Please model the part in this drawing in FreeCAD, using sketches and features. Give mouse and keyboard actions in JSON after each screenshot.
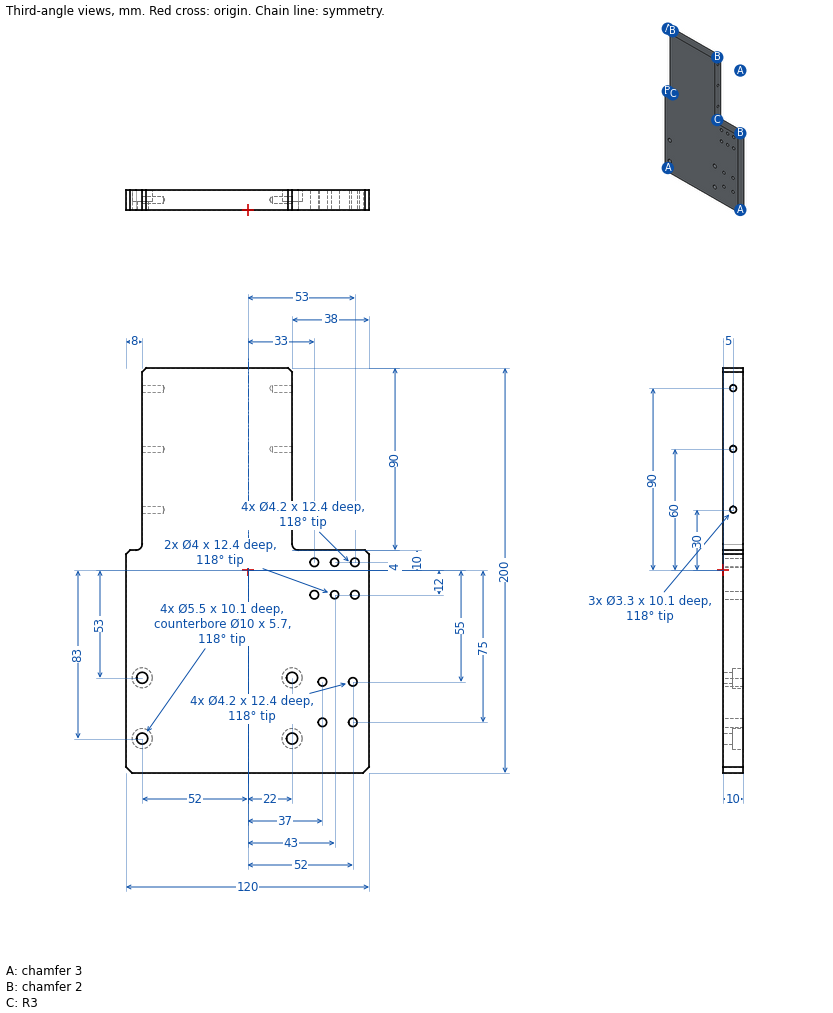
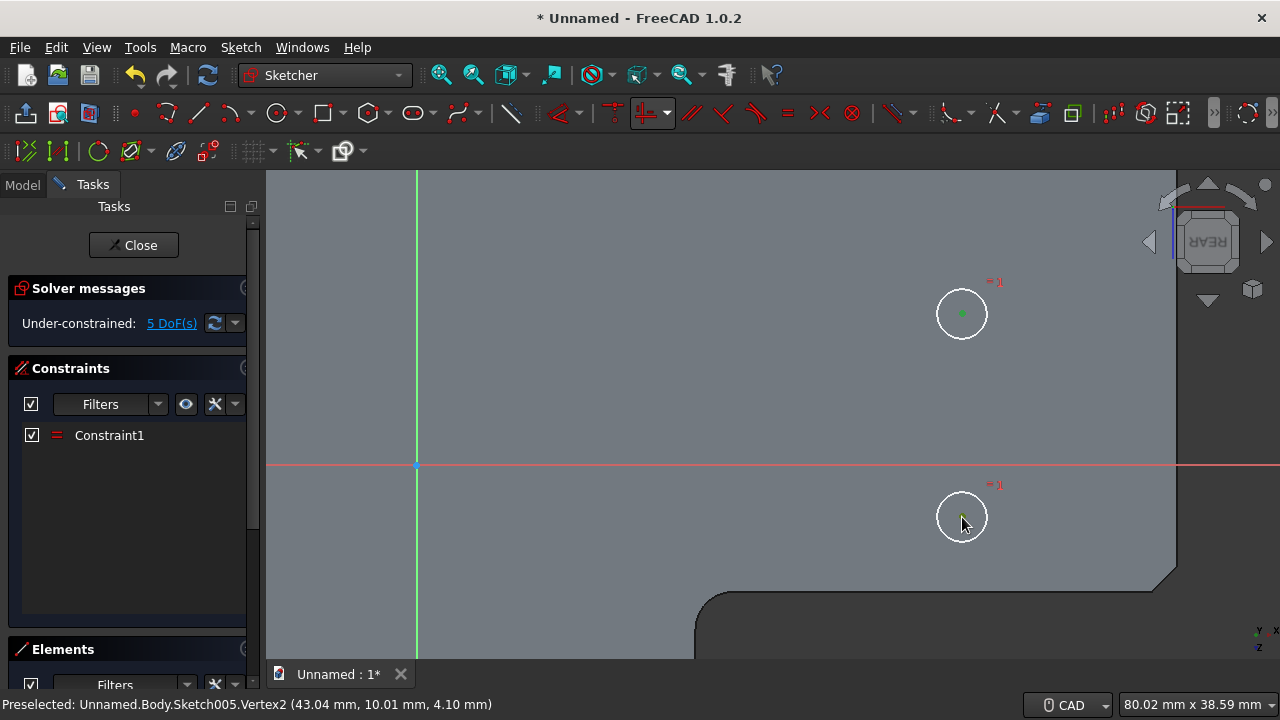
{"action": "left_click", "coordinate": [670, 114]}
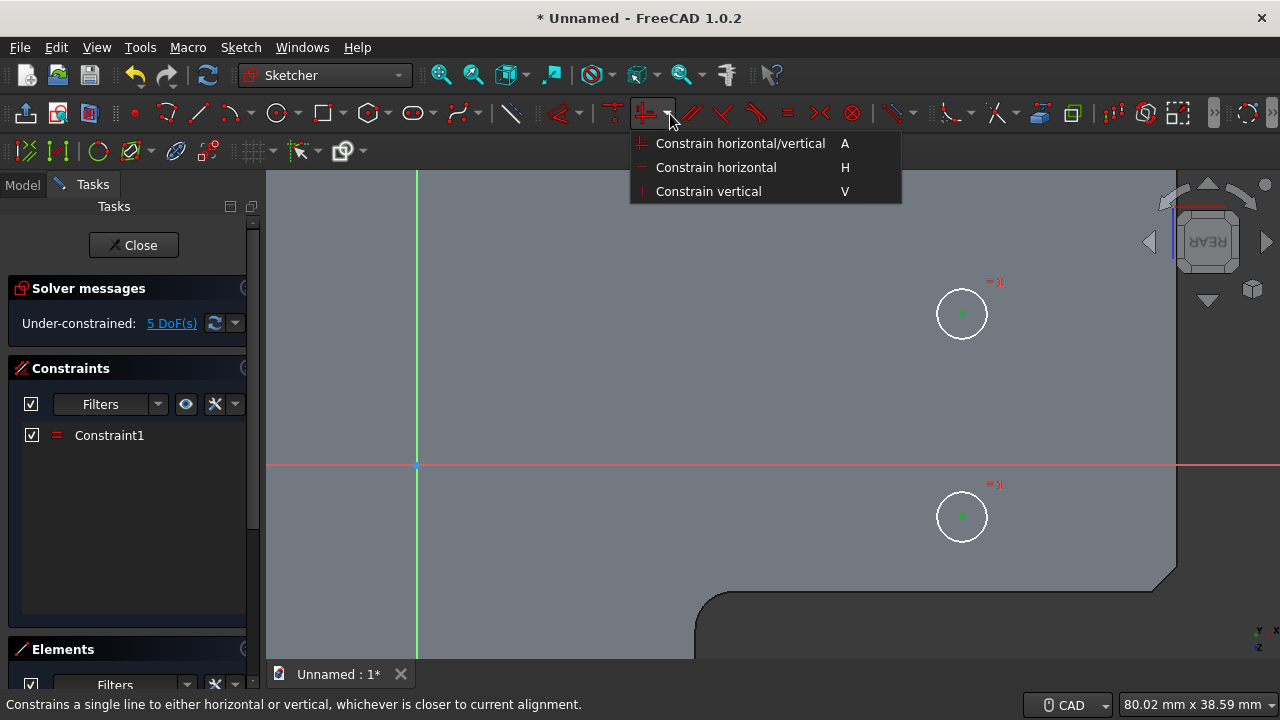
{"action": "left_click", "coordinate": [766, 191]}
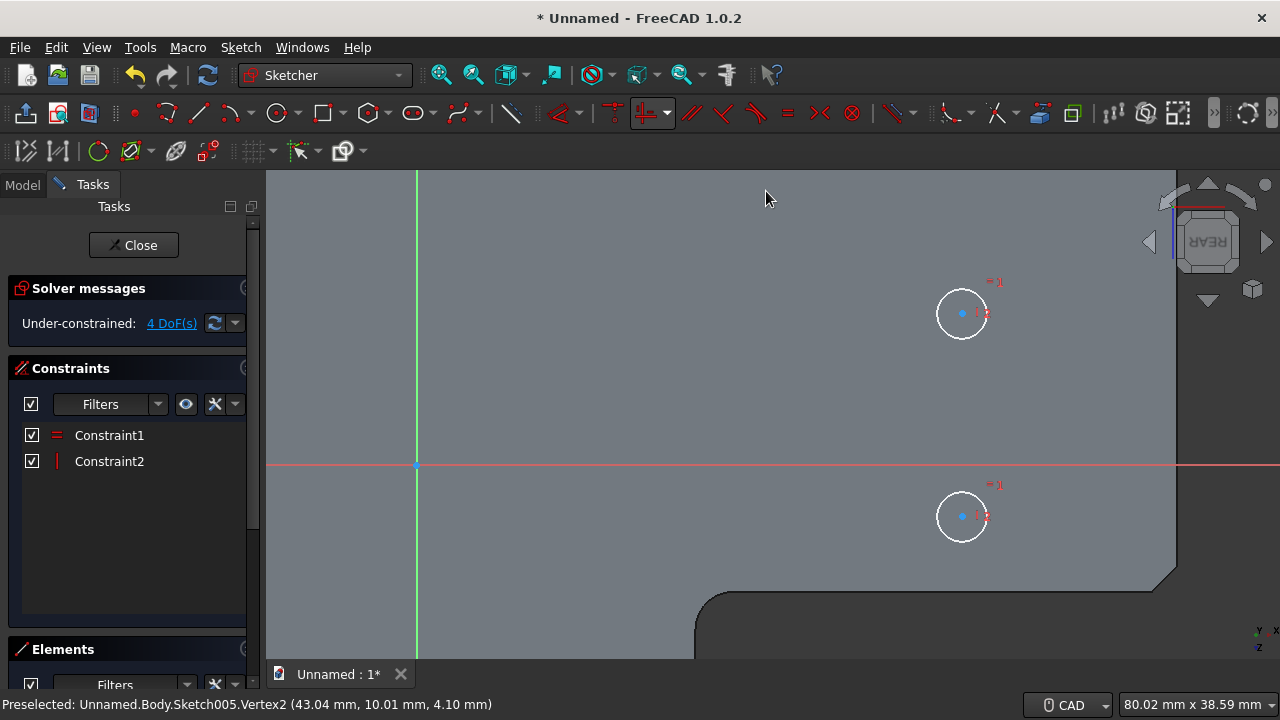
{"action": "left_click", "coordinate": [558, 114]}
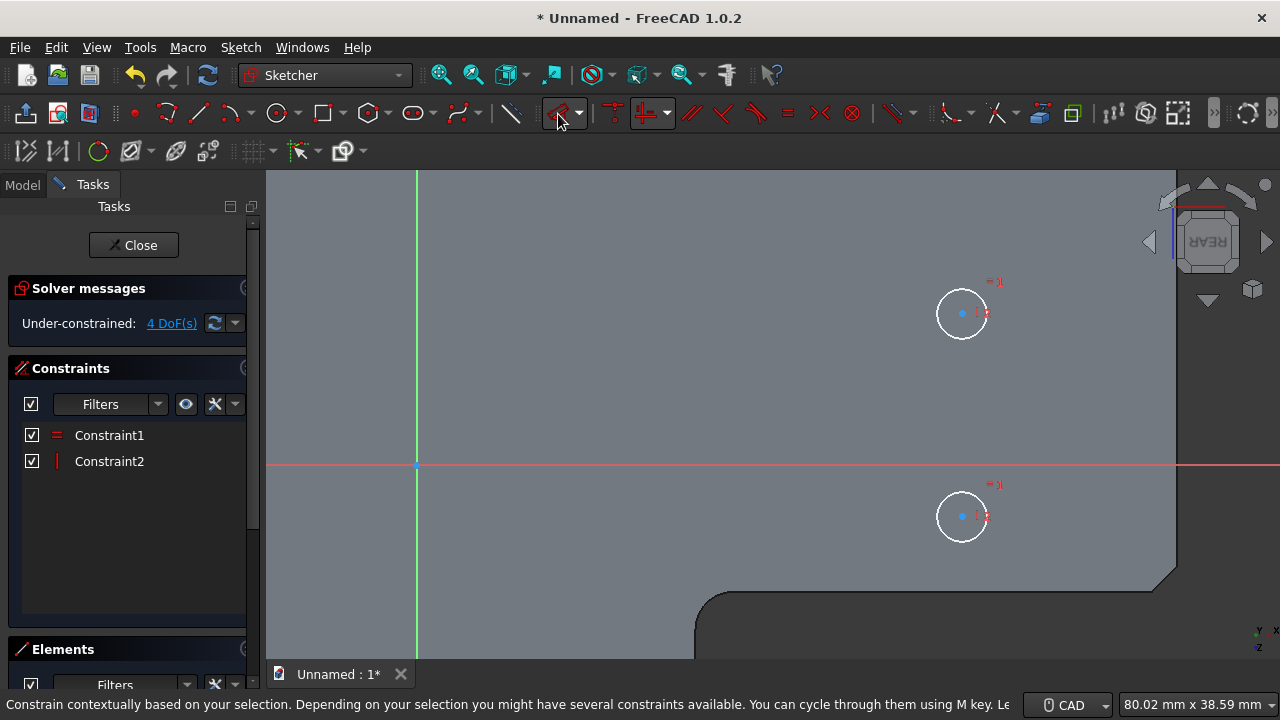
{"action": "left_click", "coordinate": [979, 296]}
{"action": "left_click", "coordinate": [1001, 273]}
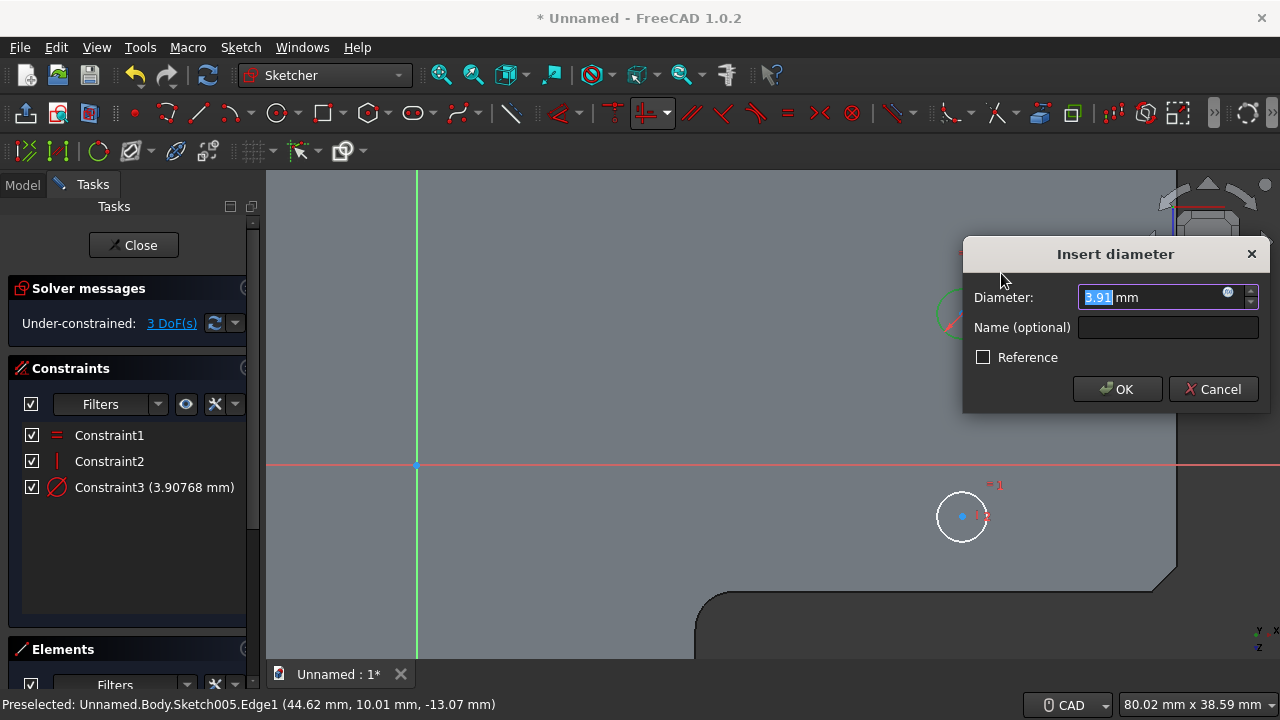
{"action": "type", "text": "4"}
{"action": "key", "text": "Return"}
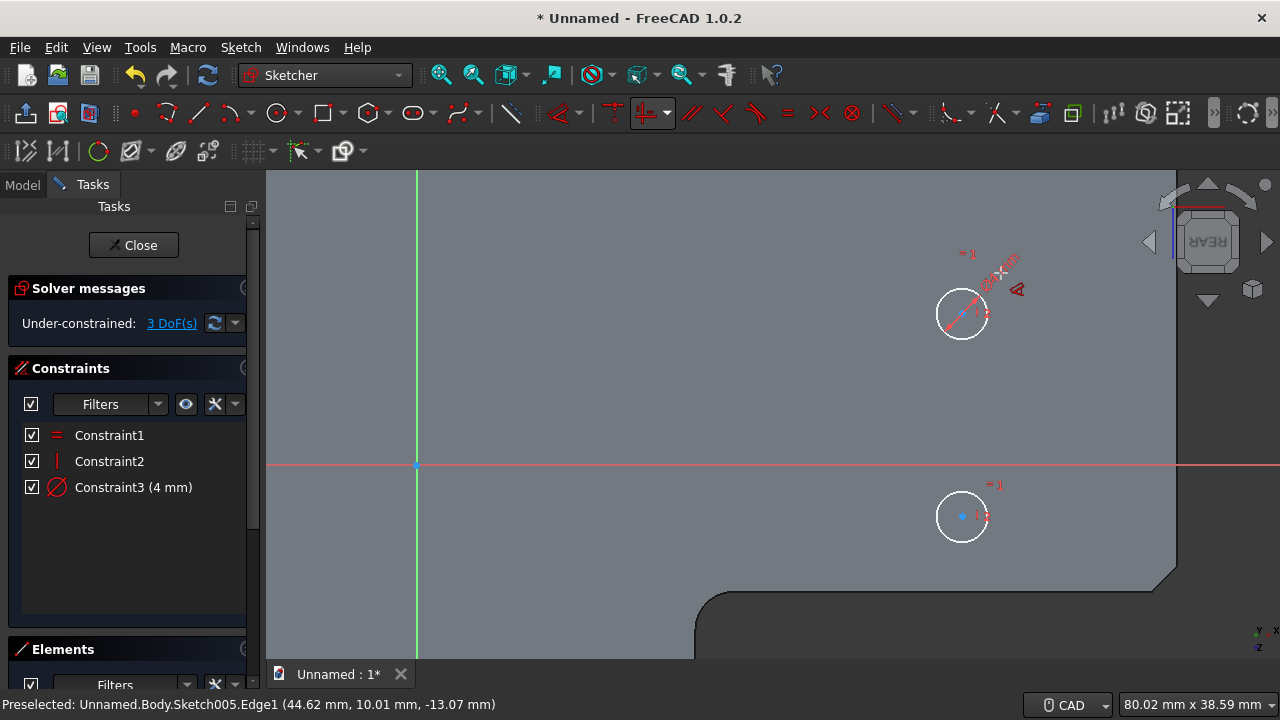
{"action": "left_click", "coordinate": [962, 517]}
{"action": "left_click", "coordinate": [383, 491]}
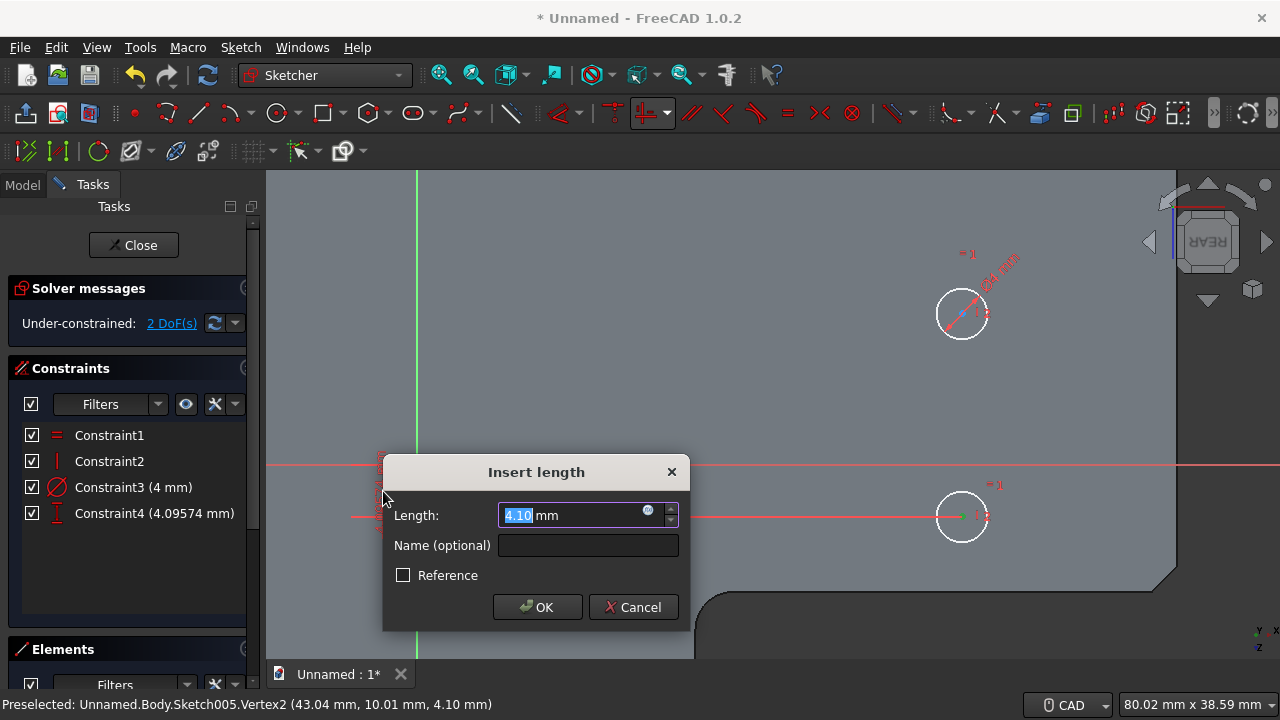
{"action": "type", "text": "4"}
{"action": "key", "text": "Return"}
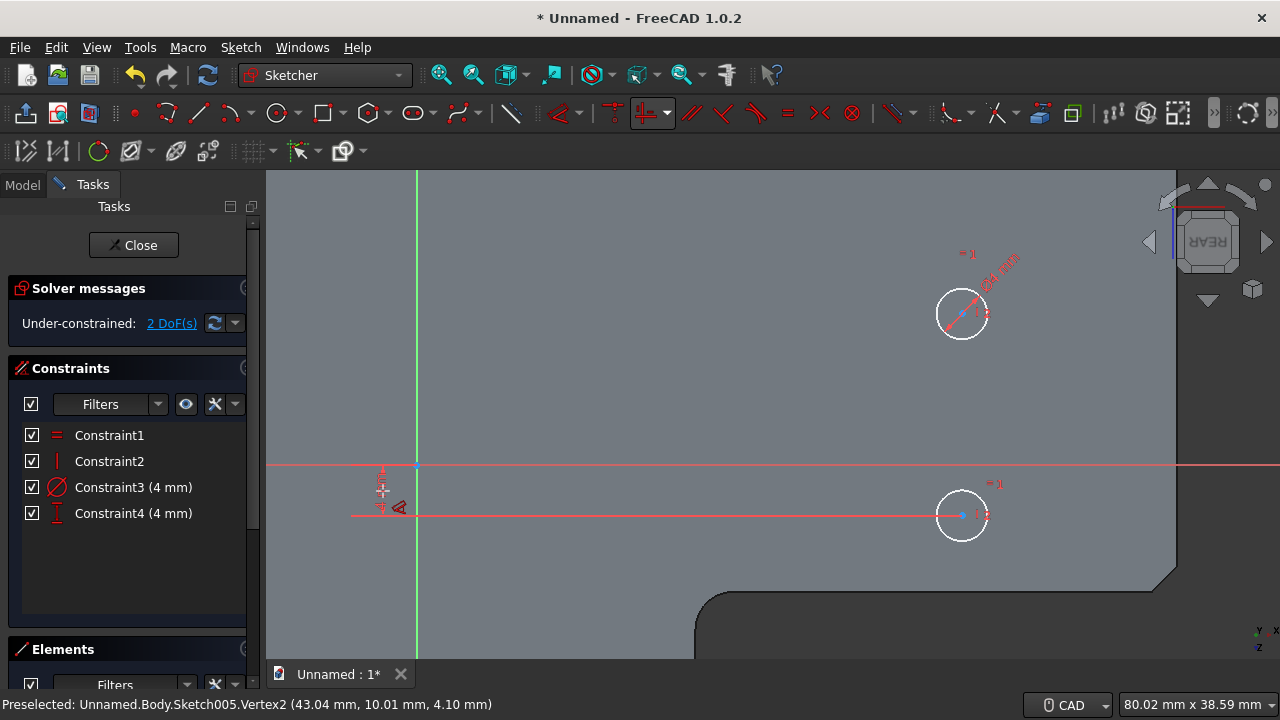
{"action": "left_click", "coordinate": [962, 314]}
{"action": "left_click", "coordinate": [689, 280]}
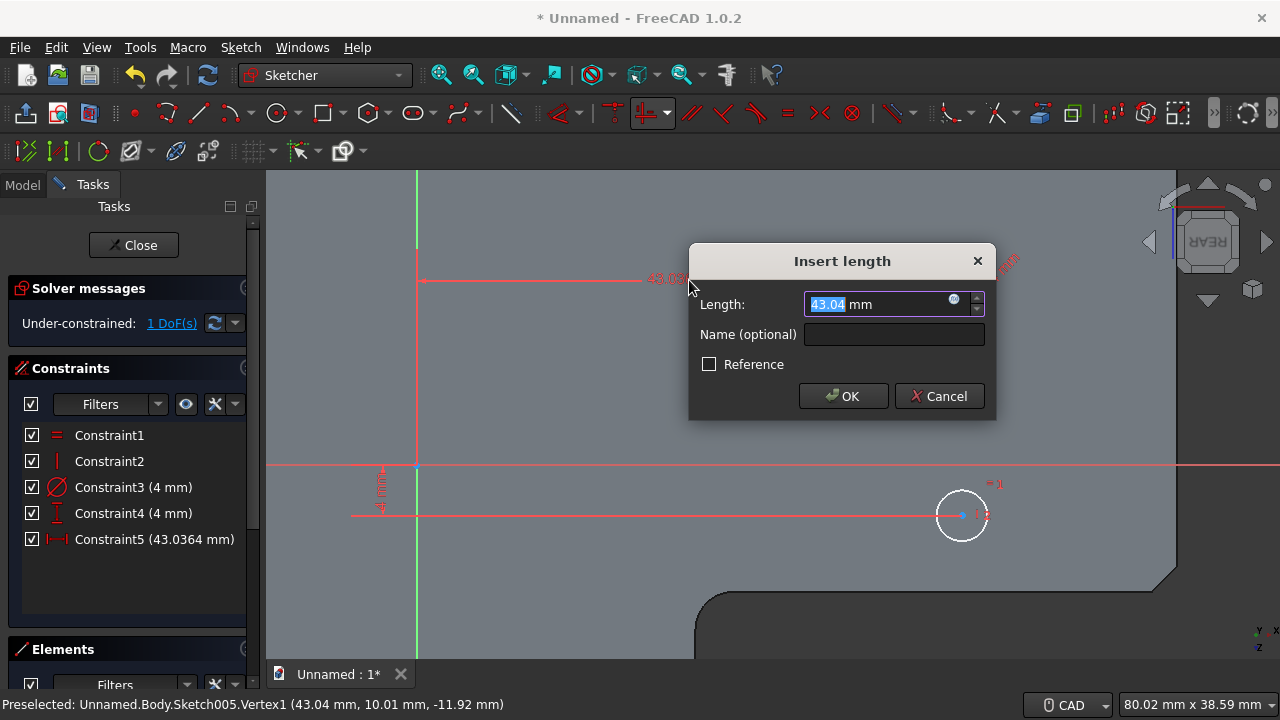
{"action": "type", "text": "43"}
{"action": "key", "text": "Return"}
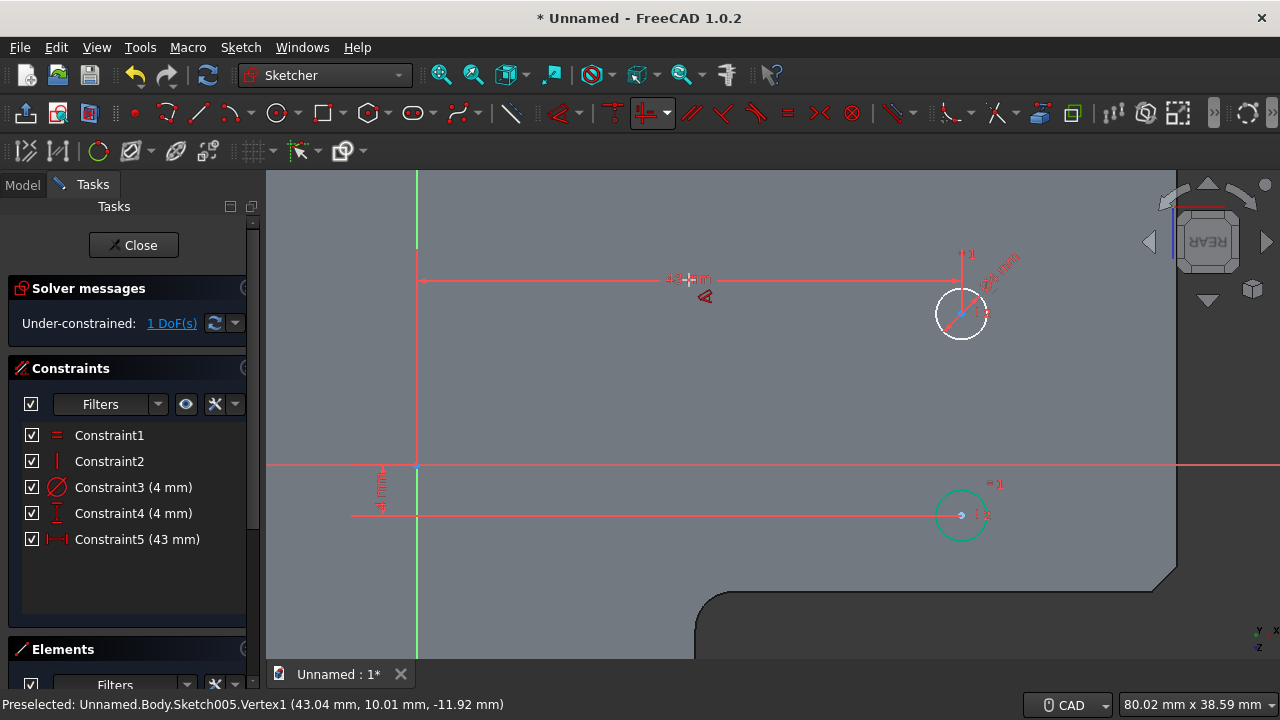
{"action": "left_click", "coordinate": [962, 314]}
{"action": "left_click", "coordinate": [383, 390]}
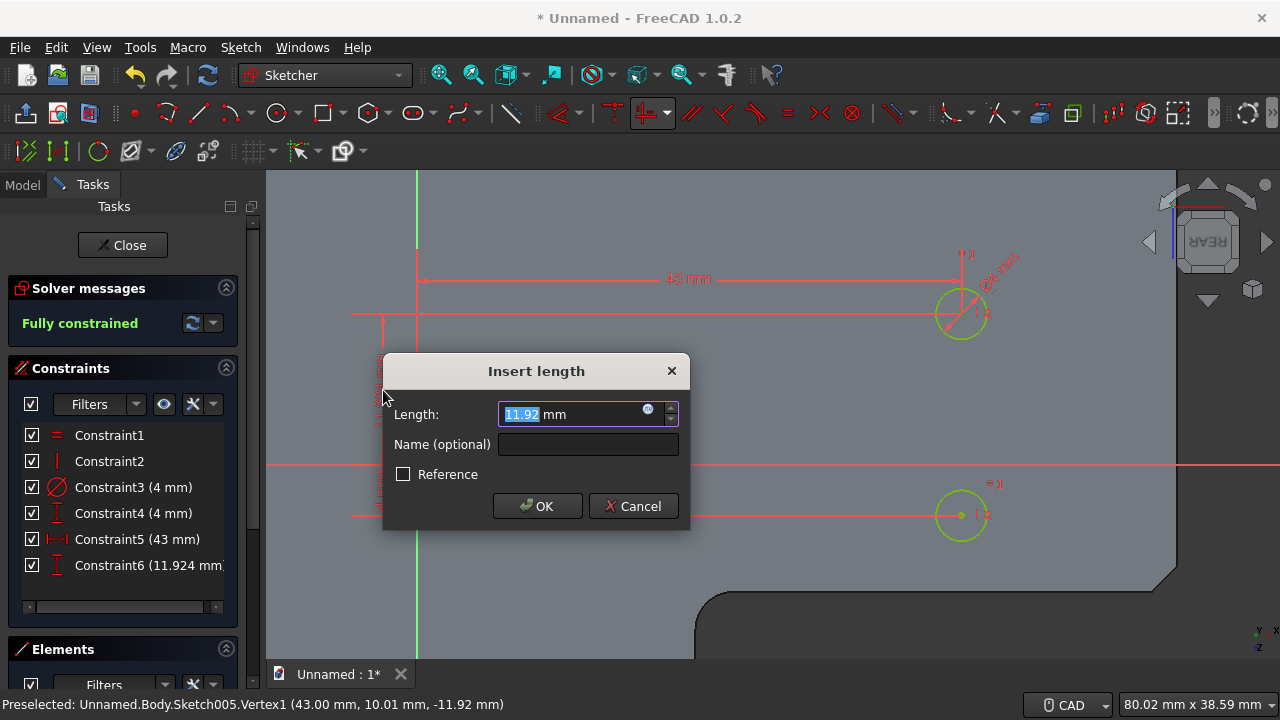
{"action": "type", "text": "12"}
{"action": "key", "text": "Return"}
{"action": "key", "text": "Escape"}